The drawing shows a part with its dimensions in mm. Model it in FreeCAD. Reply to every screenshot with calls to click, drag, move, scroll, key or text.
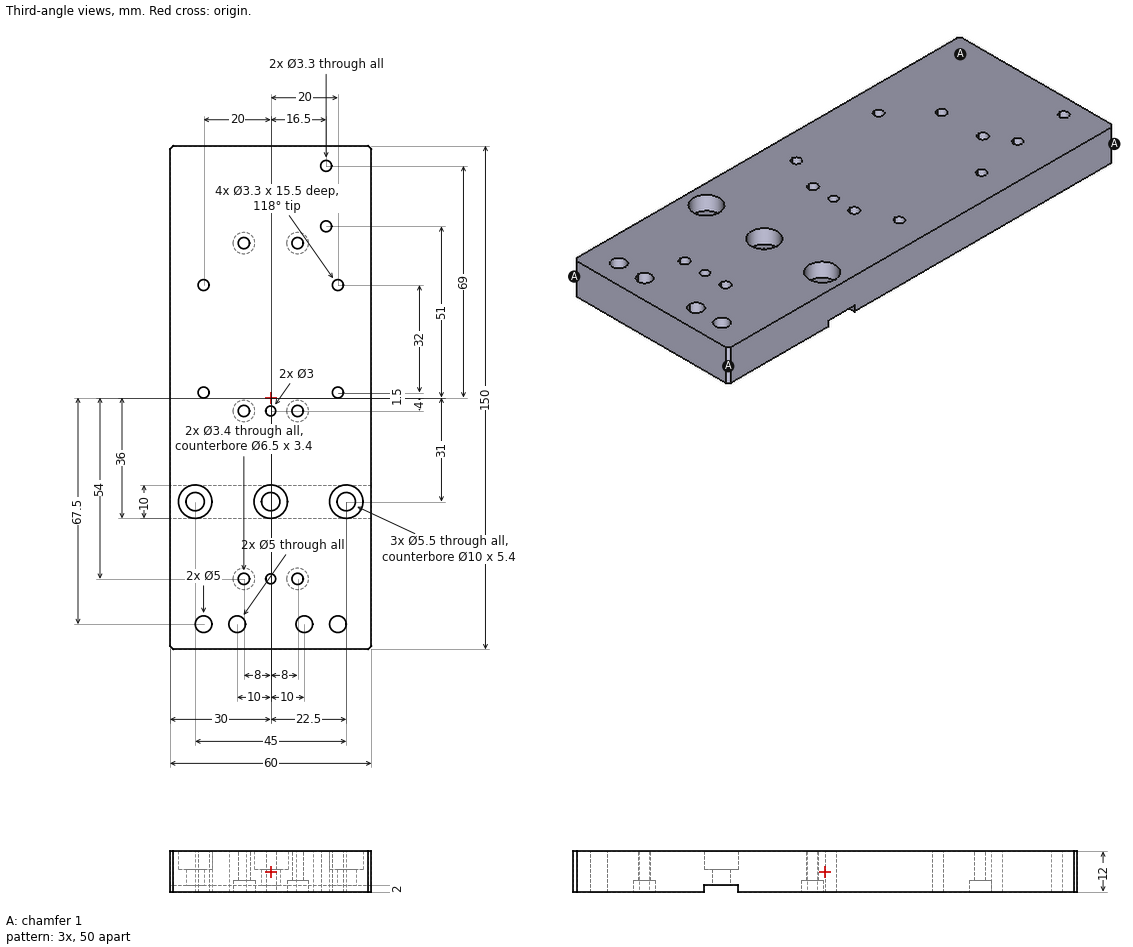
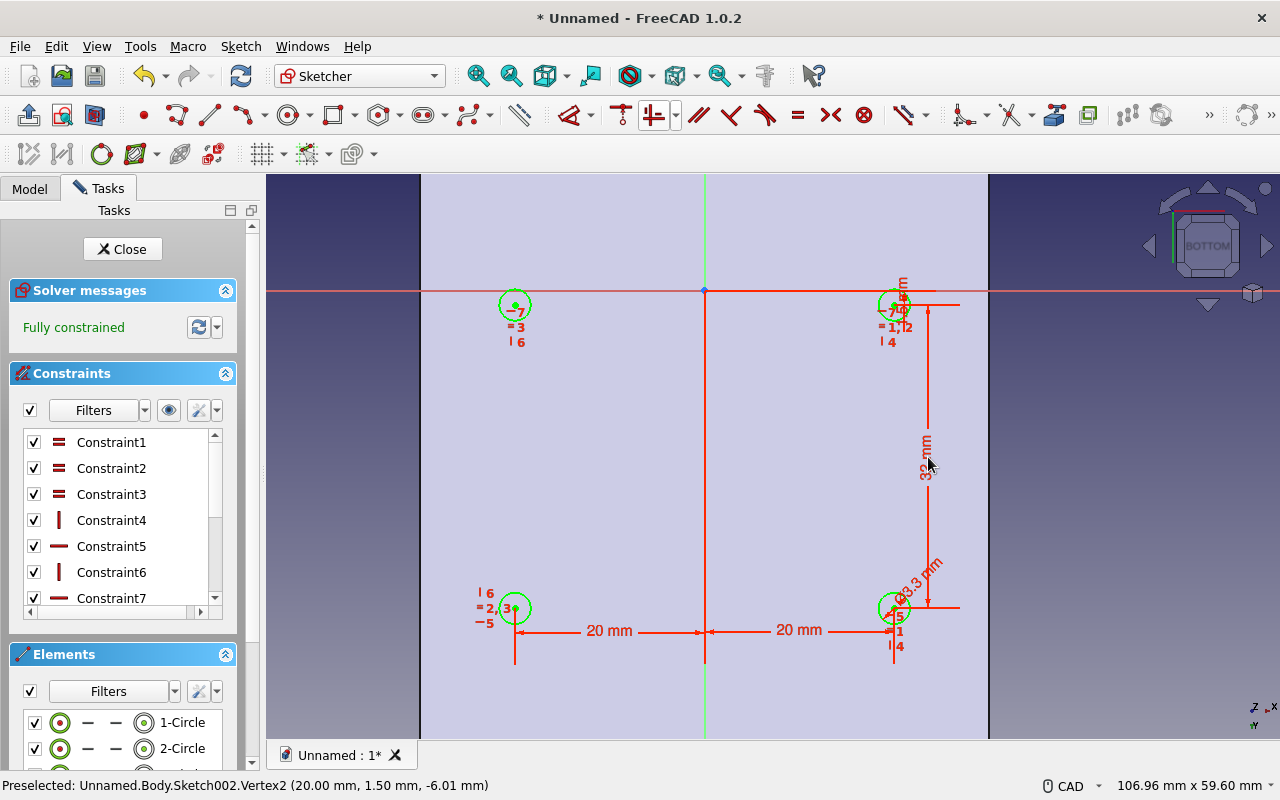
click(123, 249)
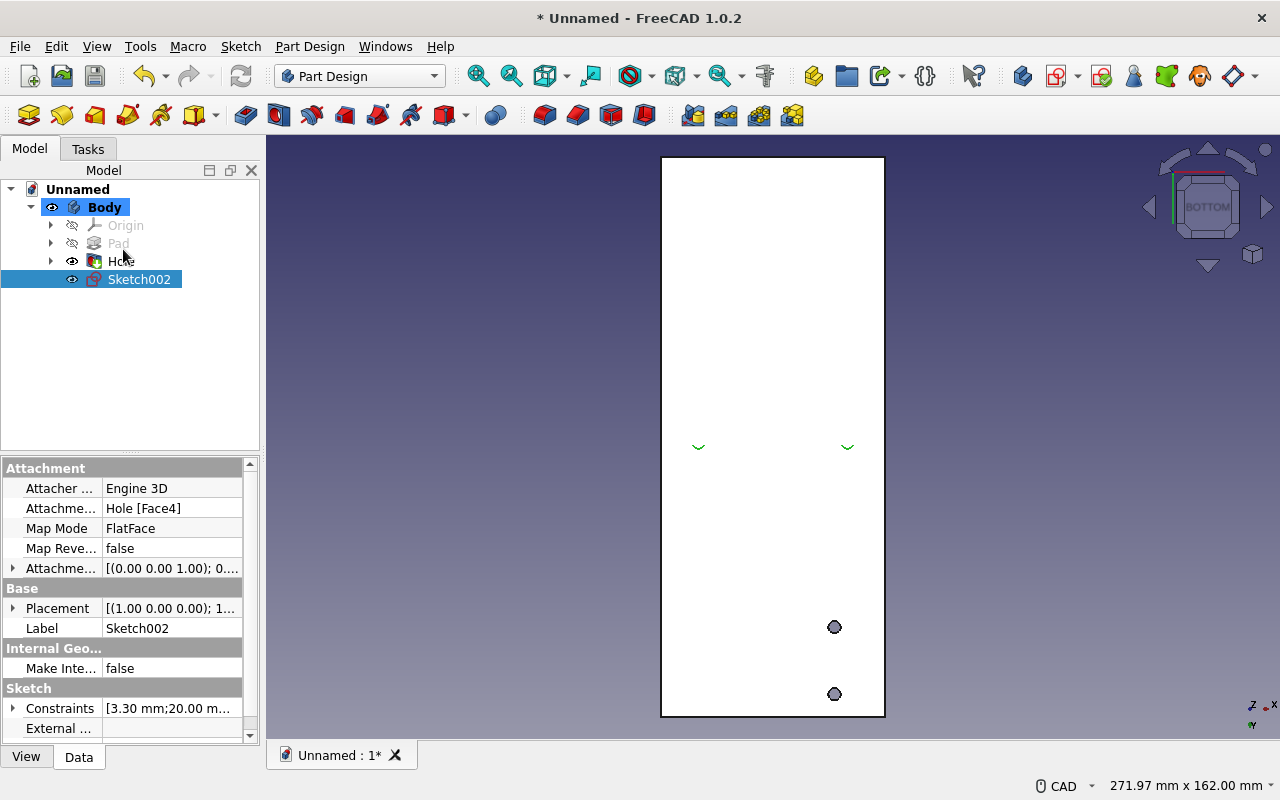
click(279, 116)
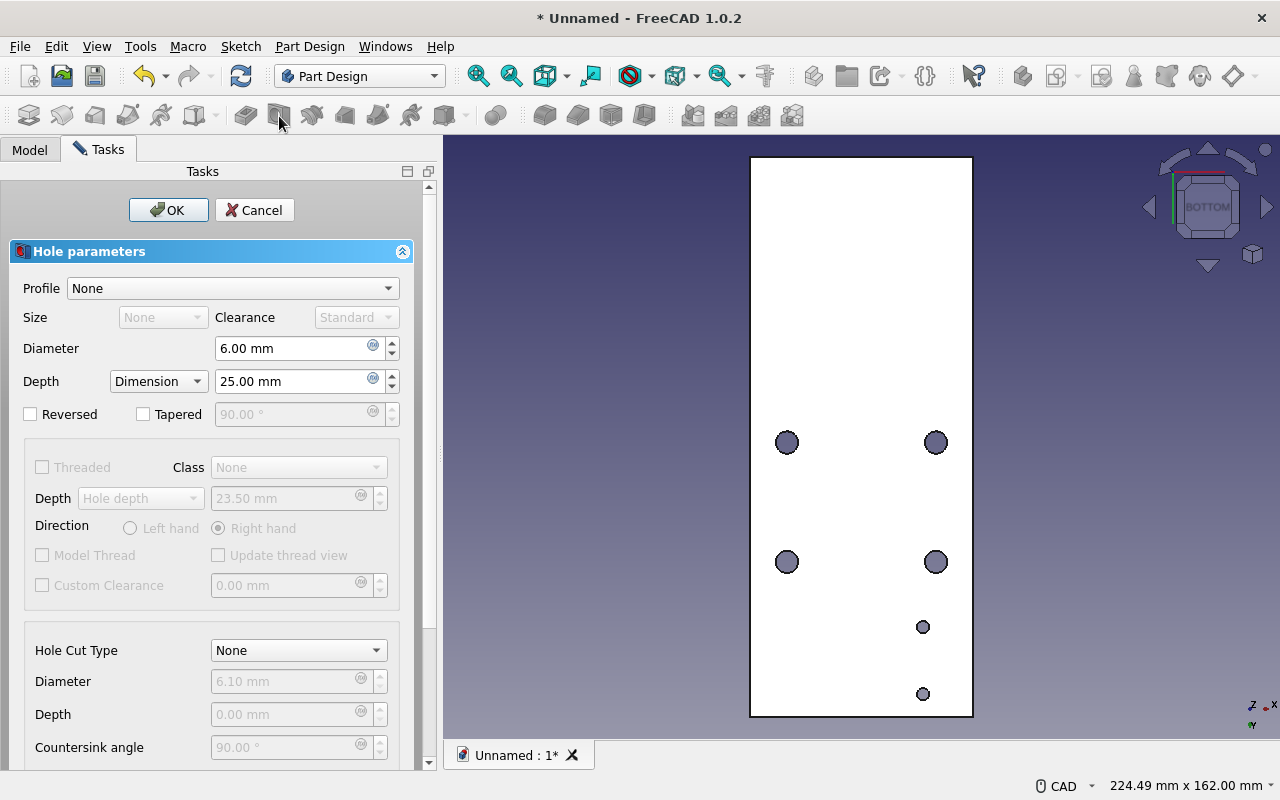
triple_click(300, 348)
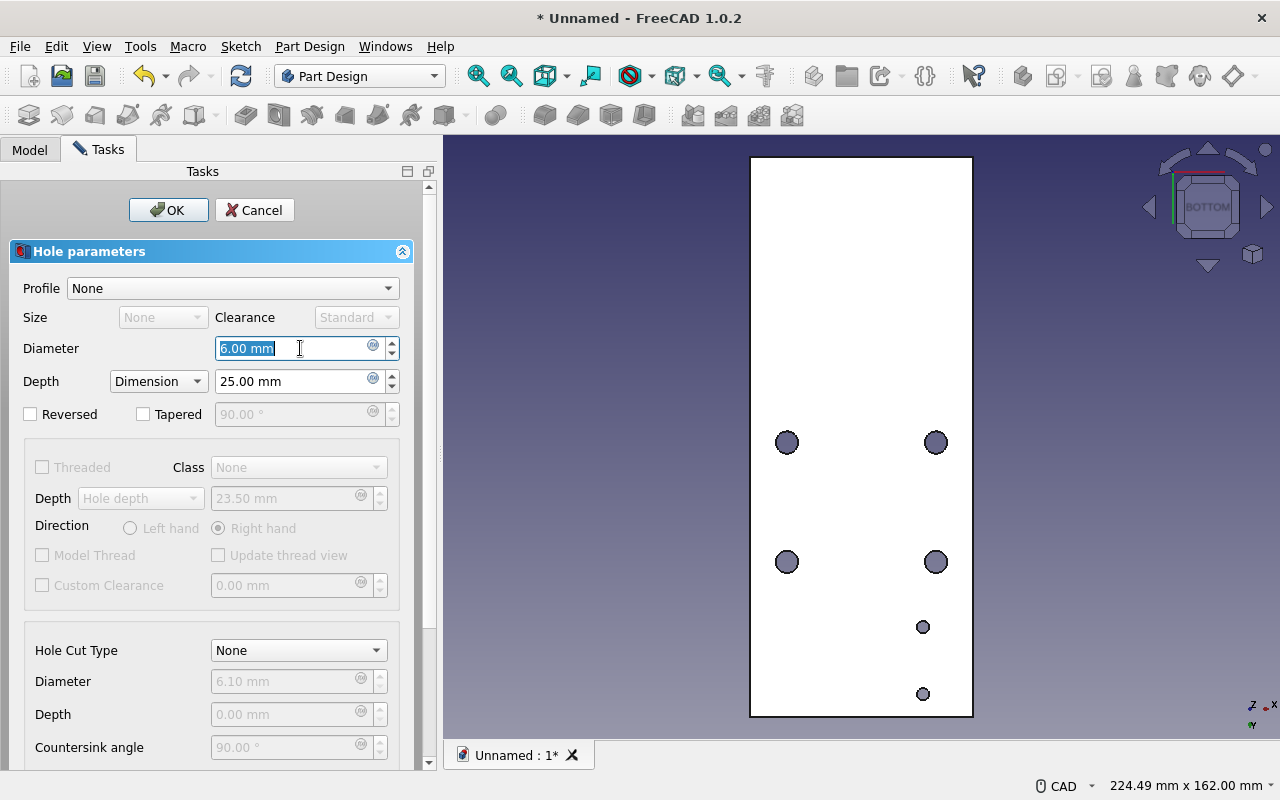
text(3.3)
key(Tab)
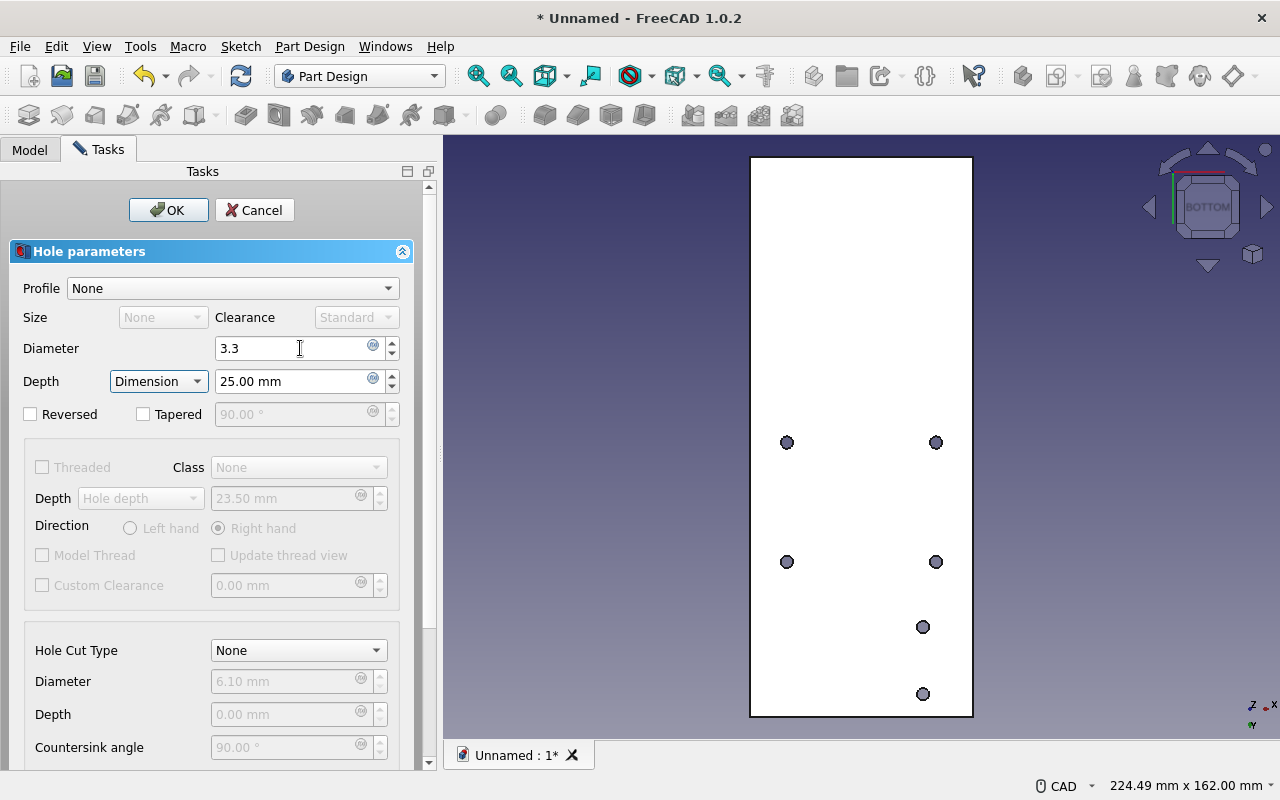
triple_click(300, 382)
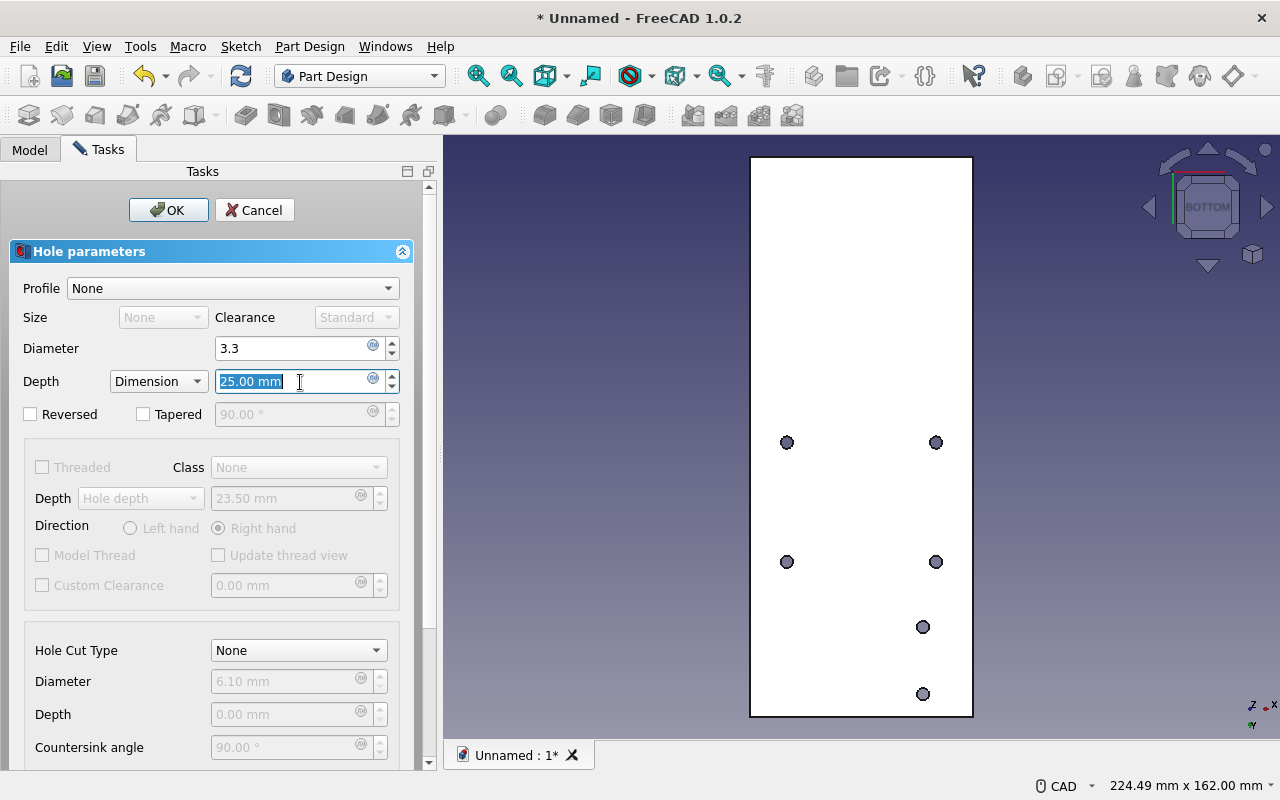
text(15.5)
key(Tab)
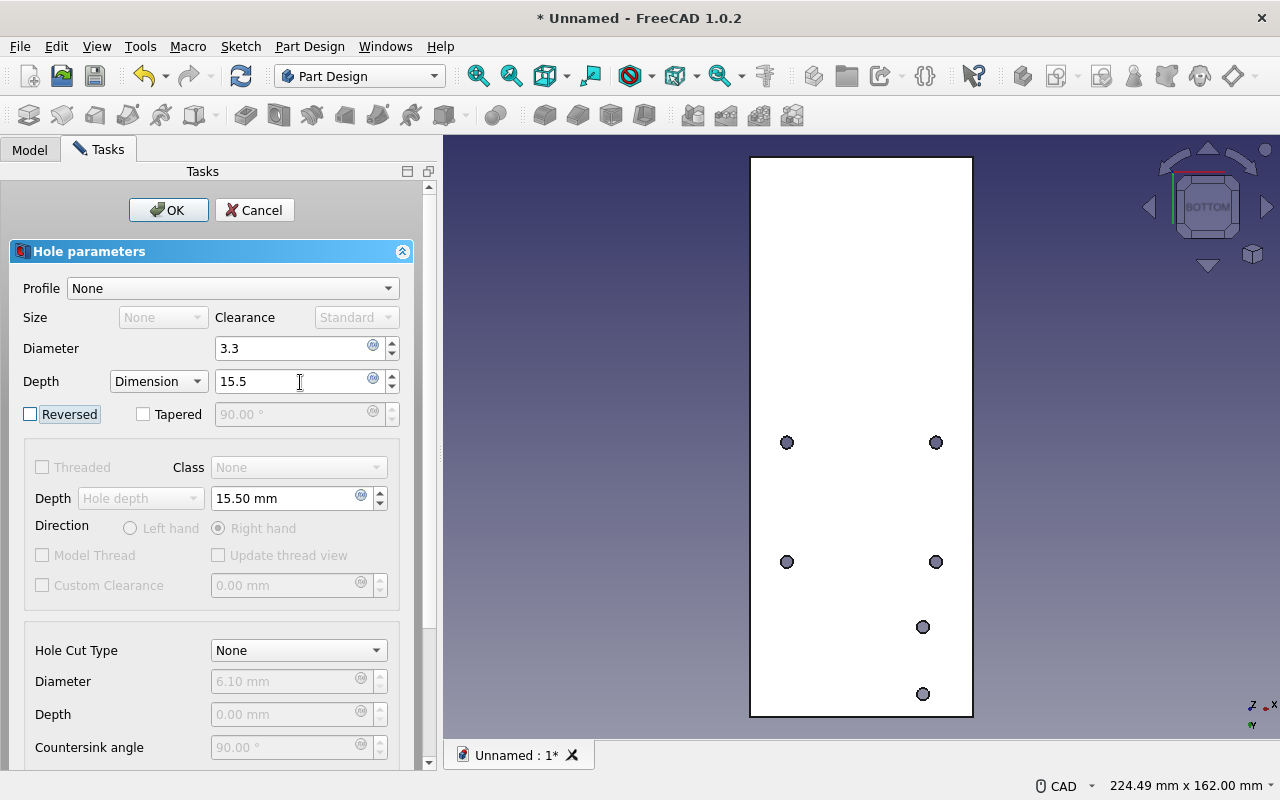
click(169, 210)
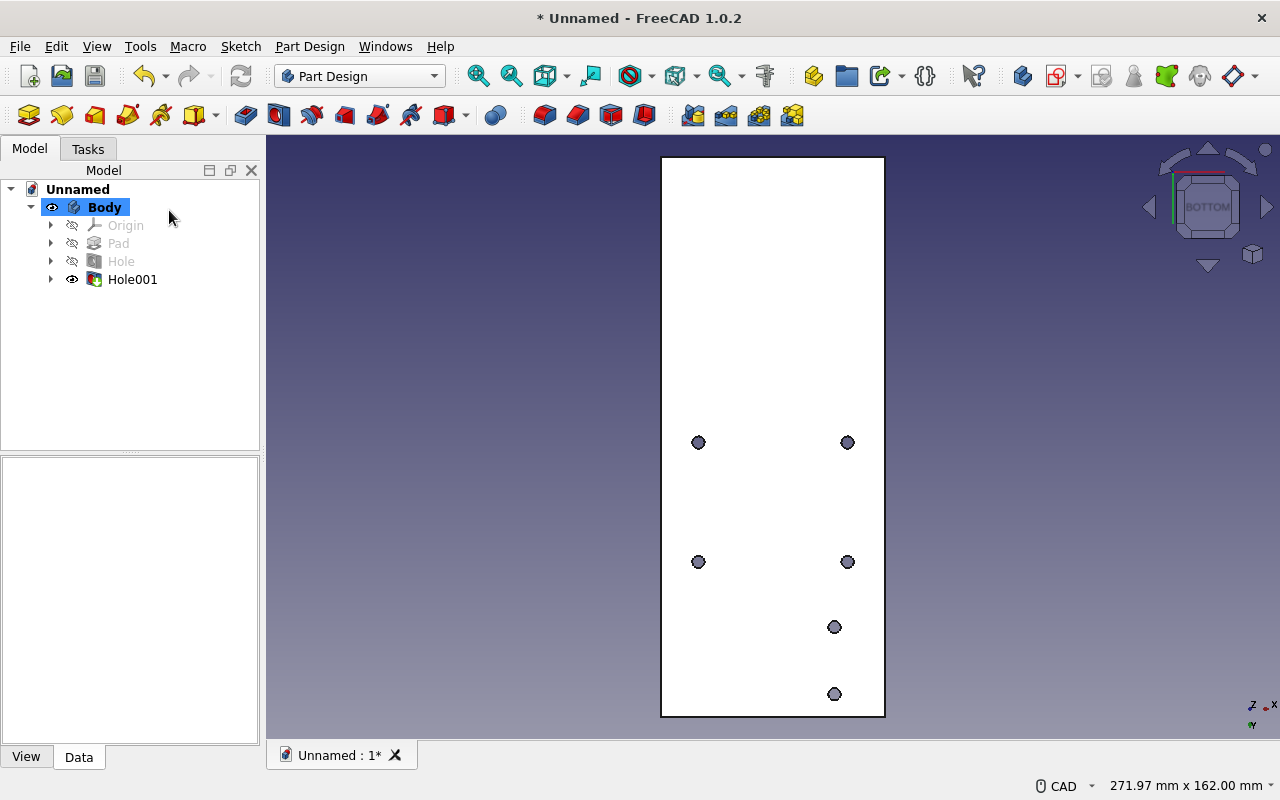
click(773, 276)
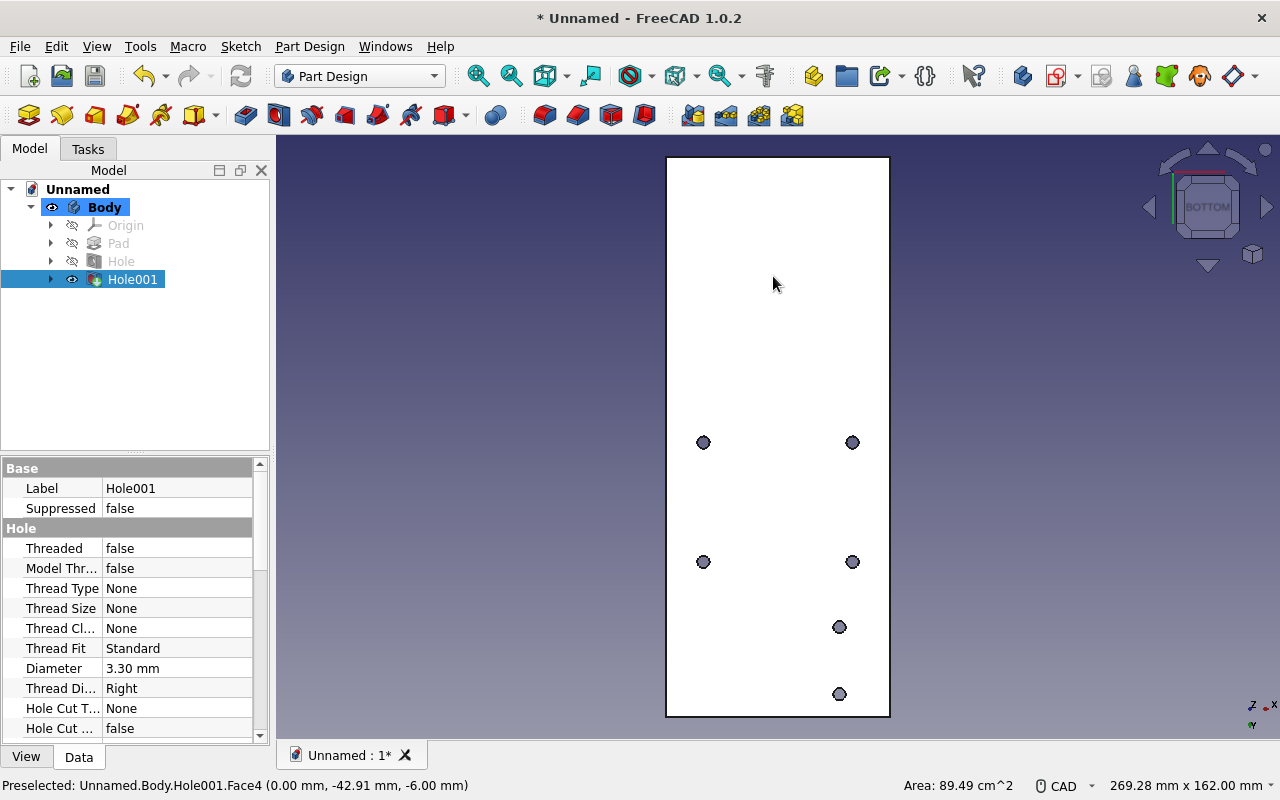
click(1056, 76)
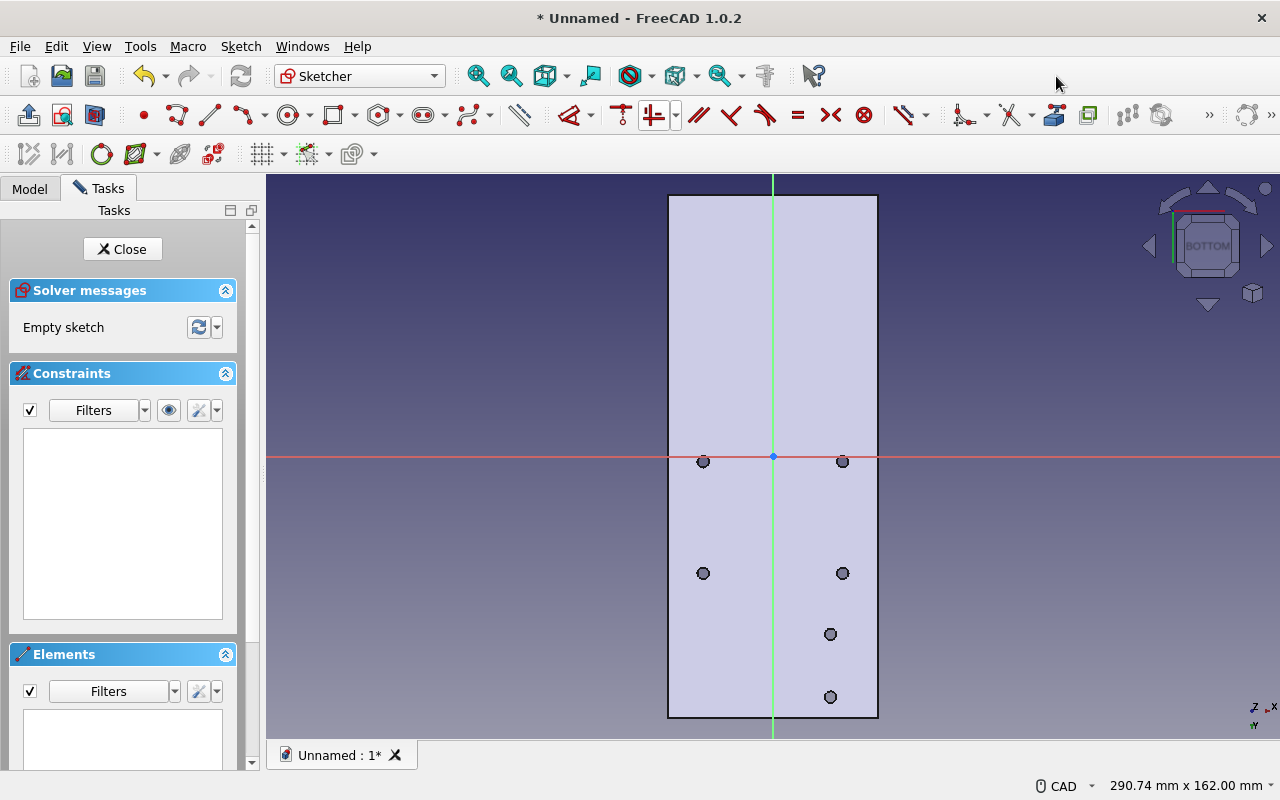
scroll(395, 711, down, 1)